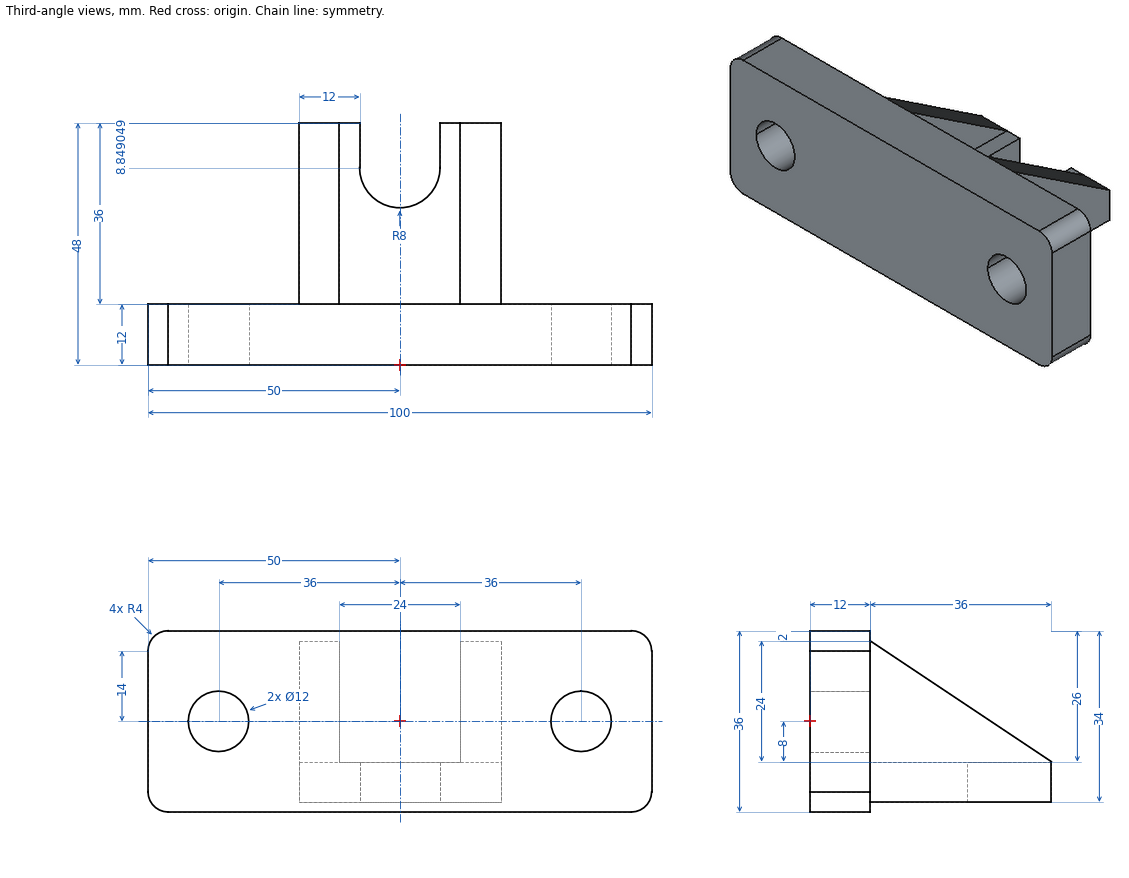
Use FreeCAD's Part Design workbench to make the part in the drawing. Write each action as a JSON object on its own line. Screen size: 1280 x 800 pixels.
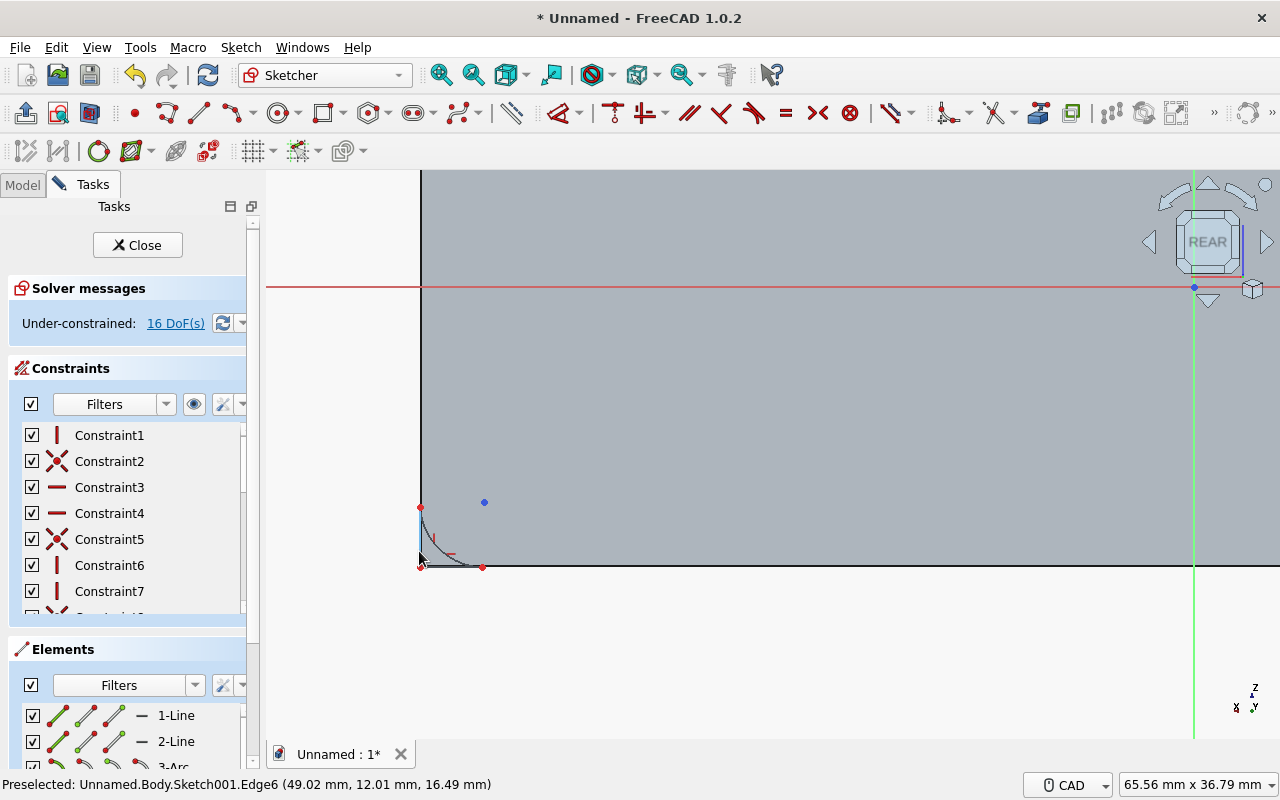
{"action": "left_click", "coordinate": [420, 550]}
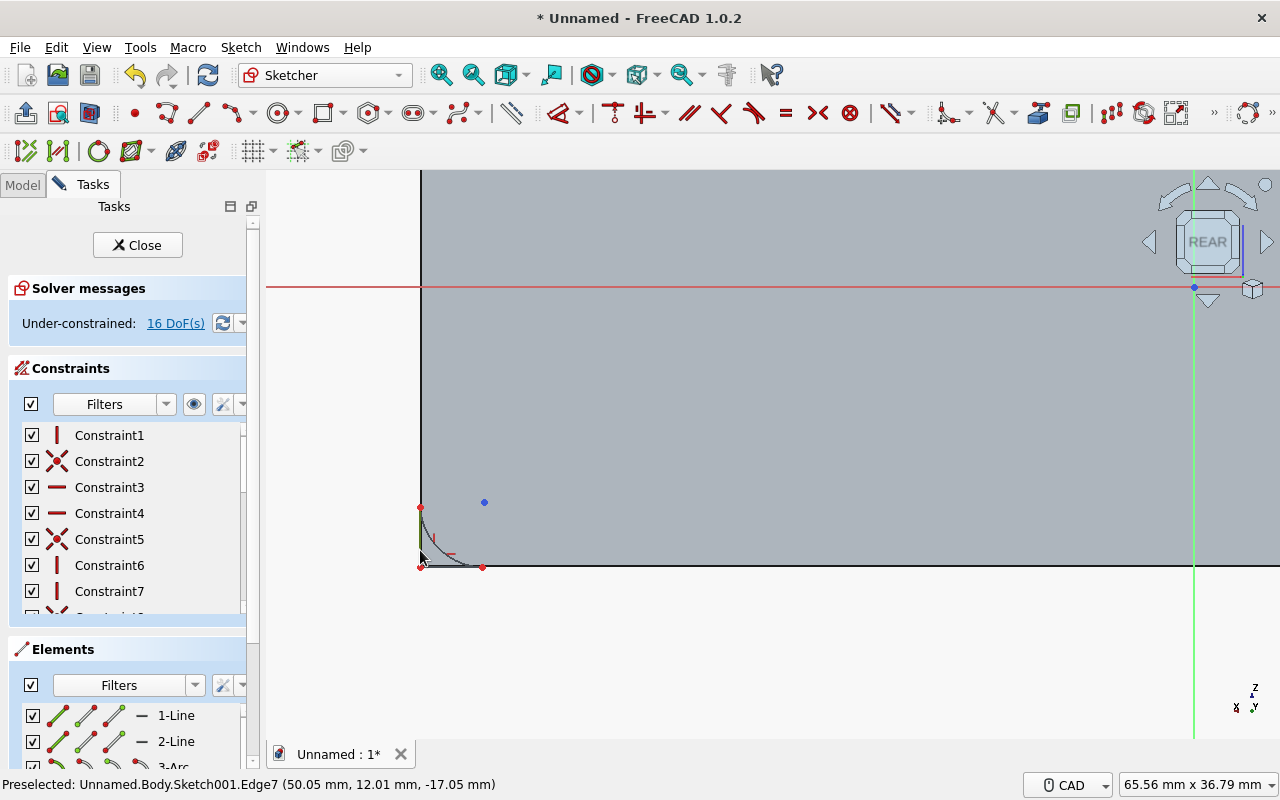
{"action": "left_click", "coordinate": [440, 549]}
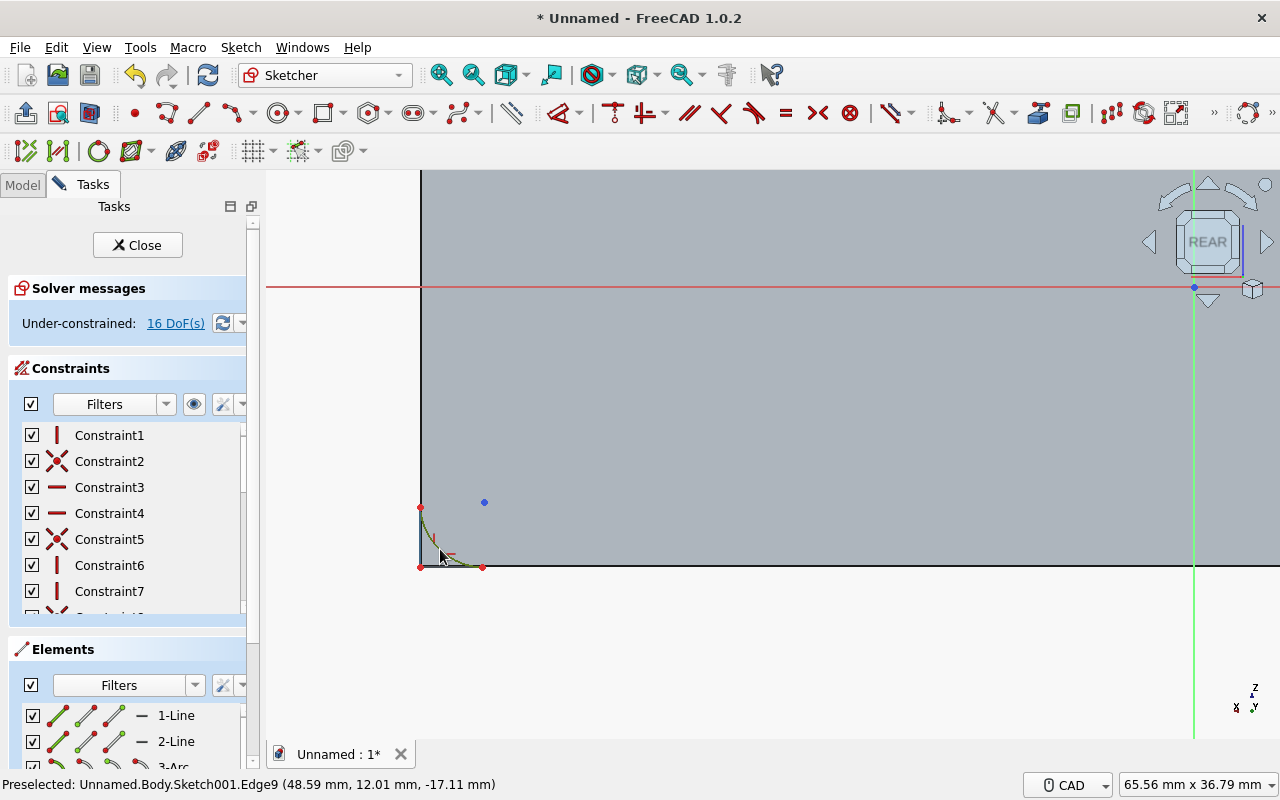
{"action": "left_click", "coordinate": [754, 114]}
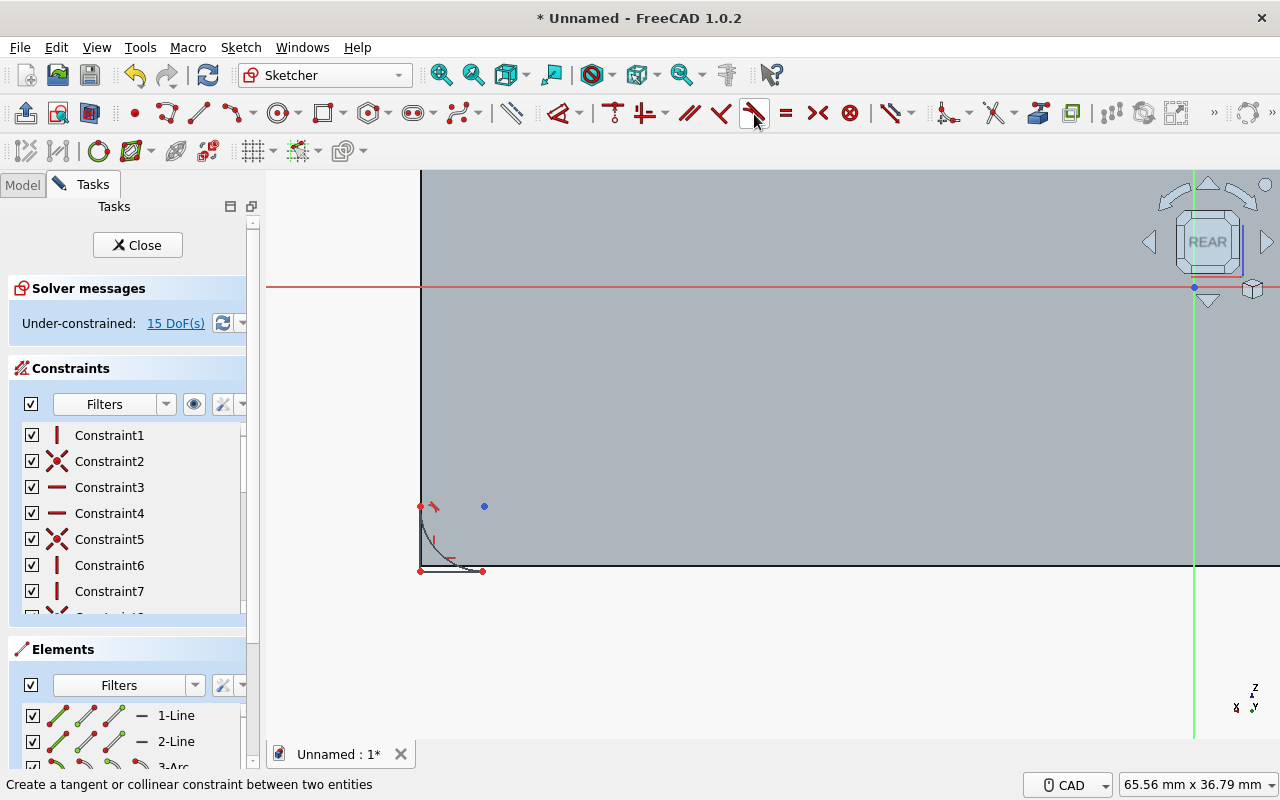
{"action": "left_click", "coordinate": [439, 572]}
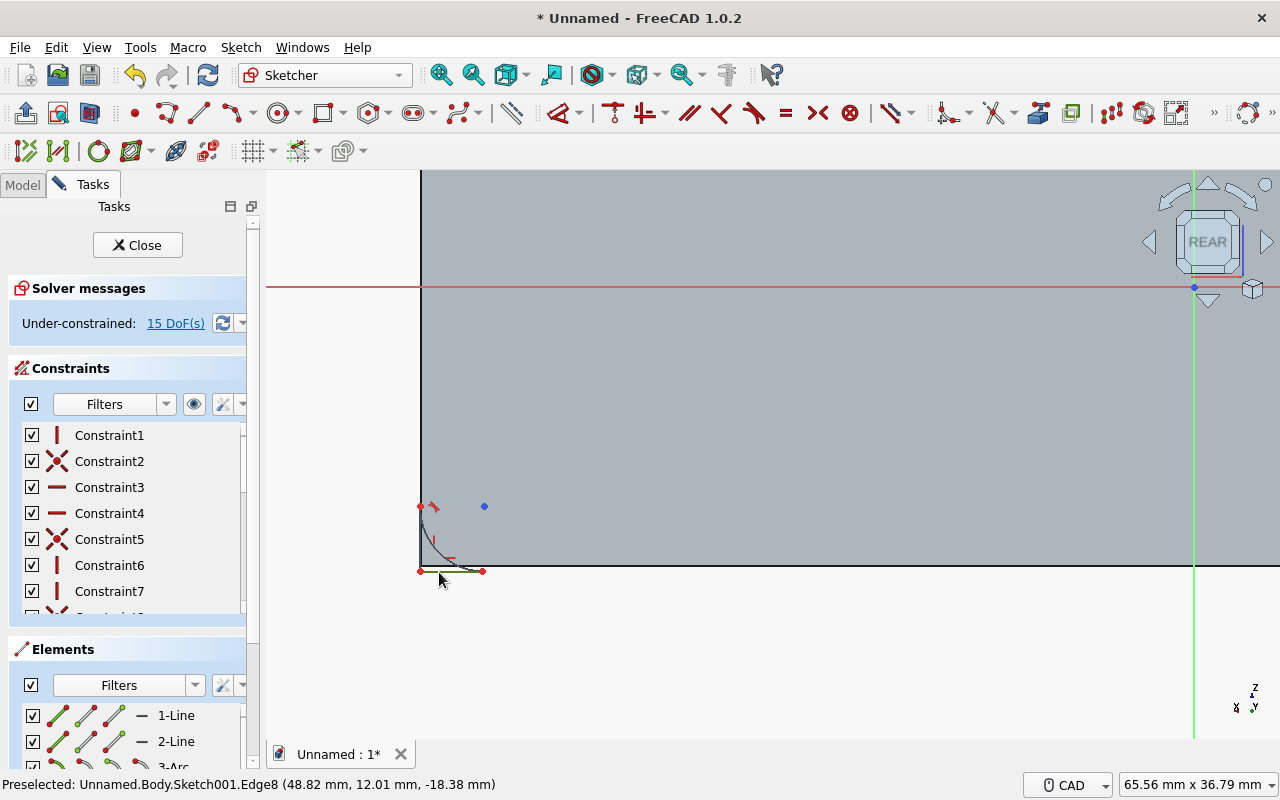
{"action": "left_click", "coordinate": [438, 552]}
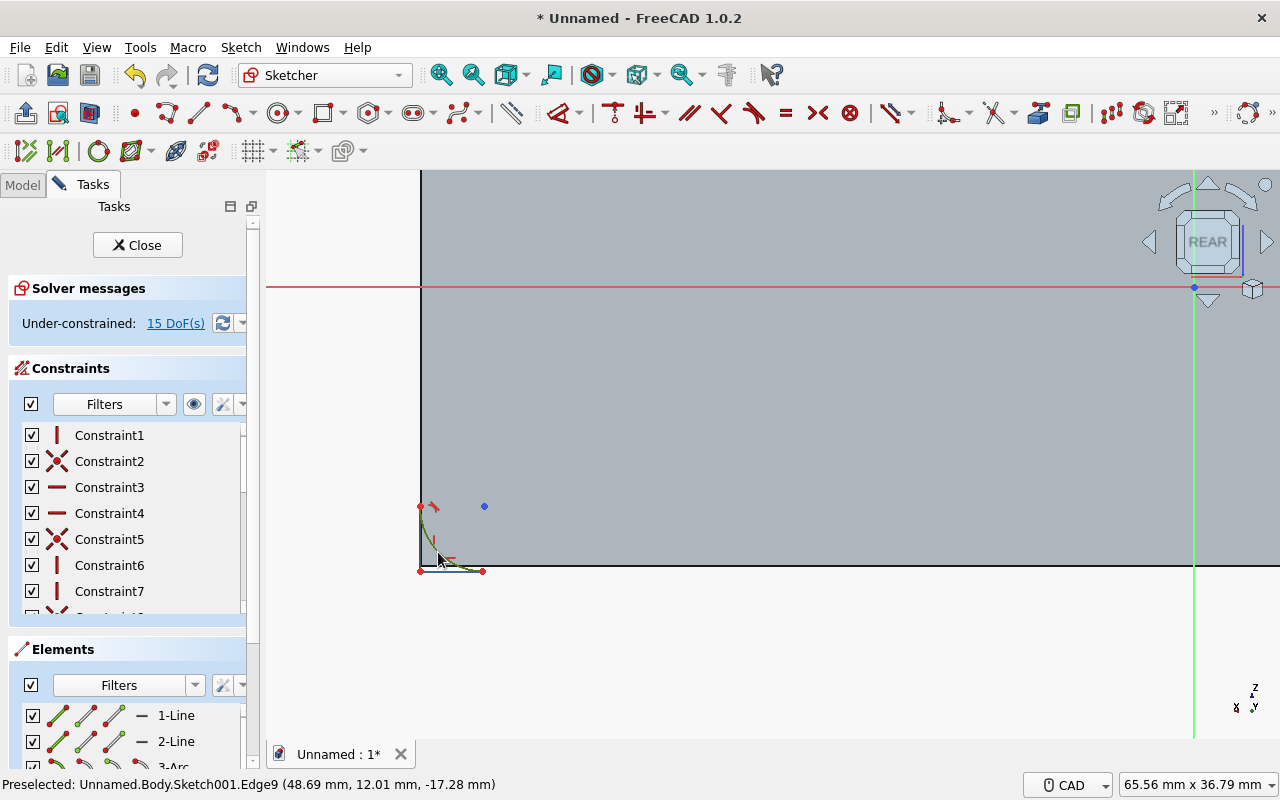
{"action": "left_click", "coordinate": [754, 114]}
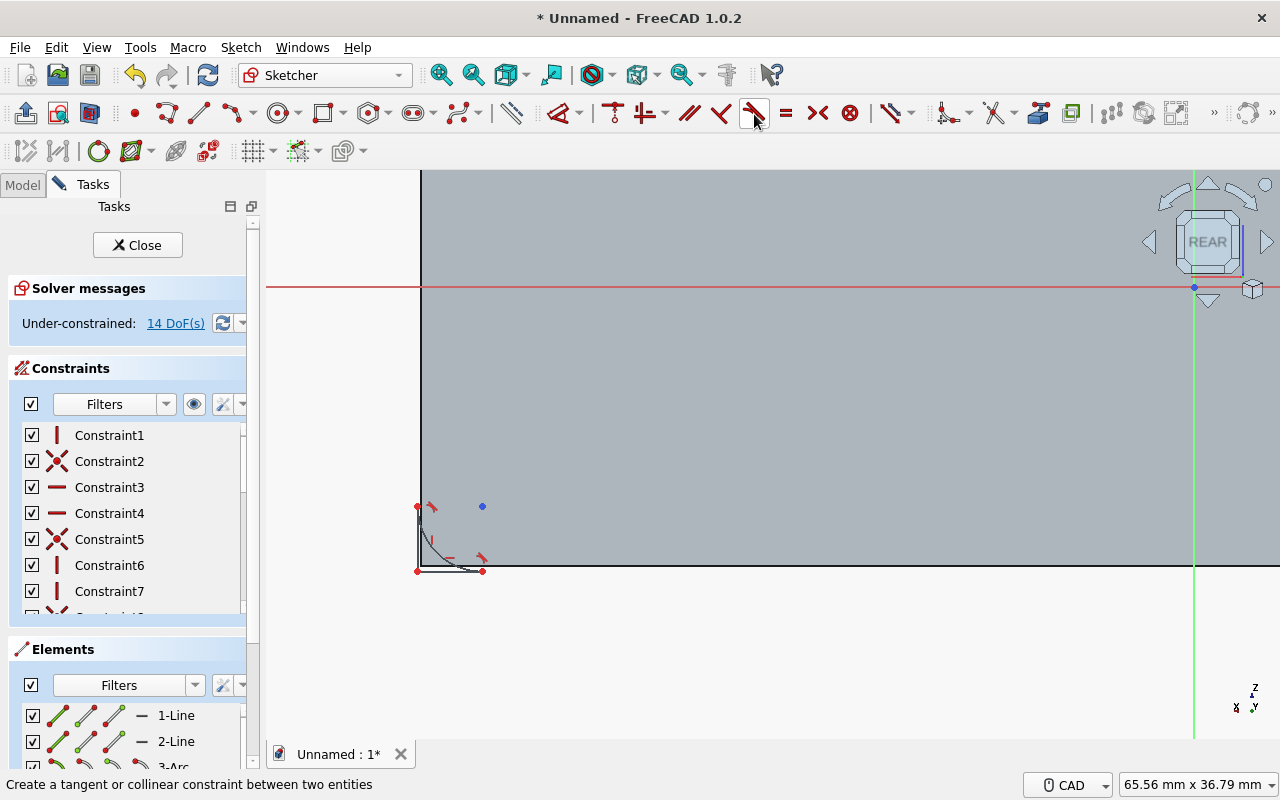
{"action": "scroll", "coordinate": [420, 552], "scroll_direction": "down", "scroll_amount": 5}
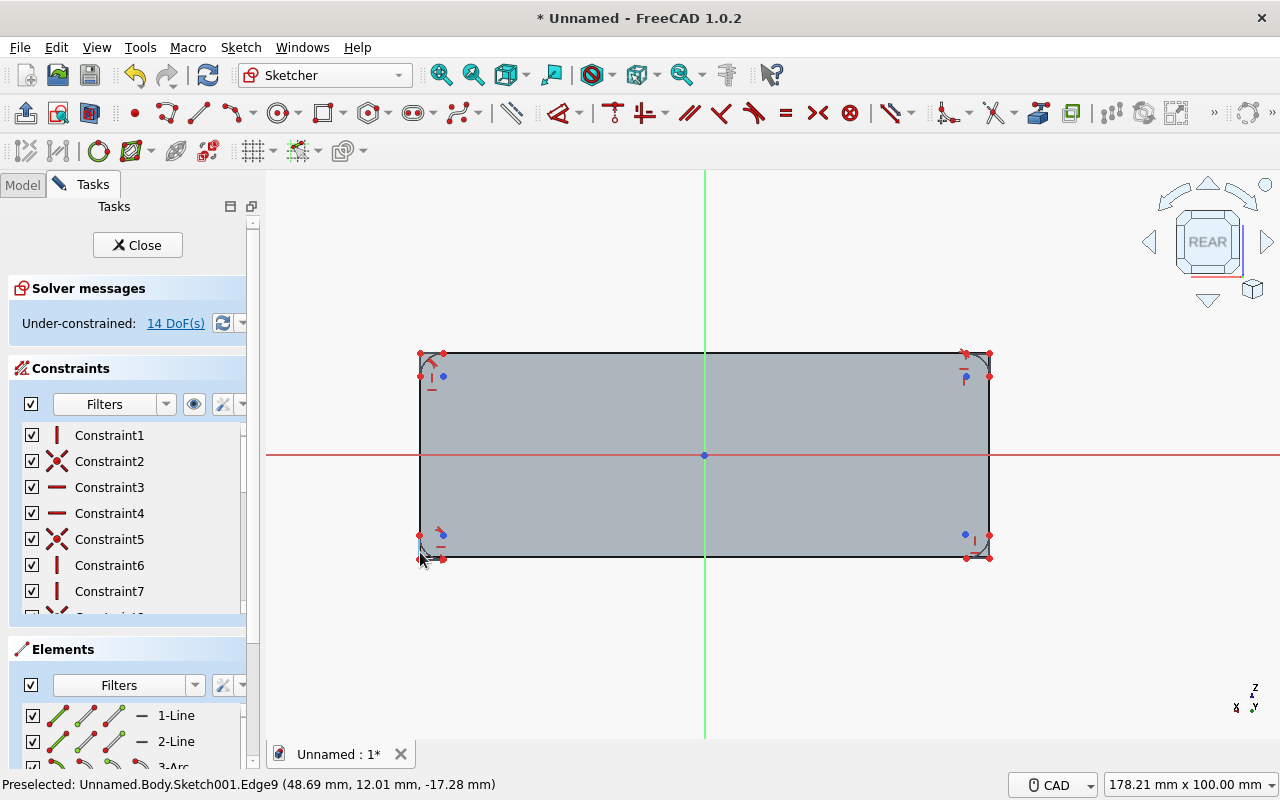
{"action": "scroll", "coordinate": [983, 558], "scroll_direction": "up", "scroll_amount": 5}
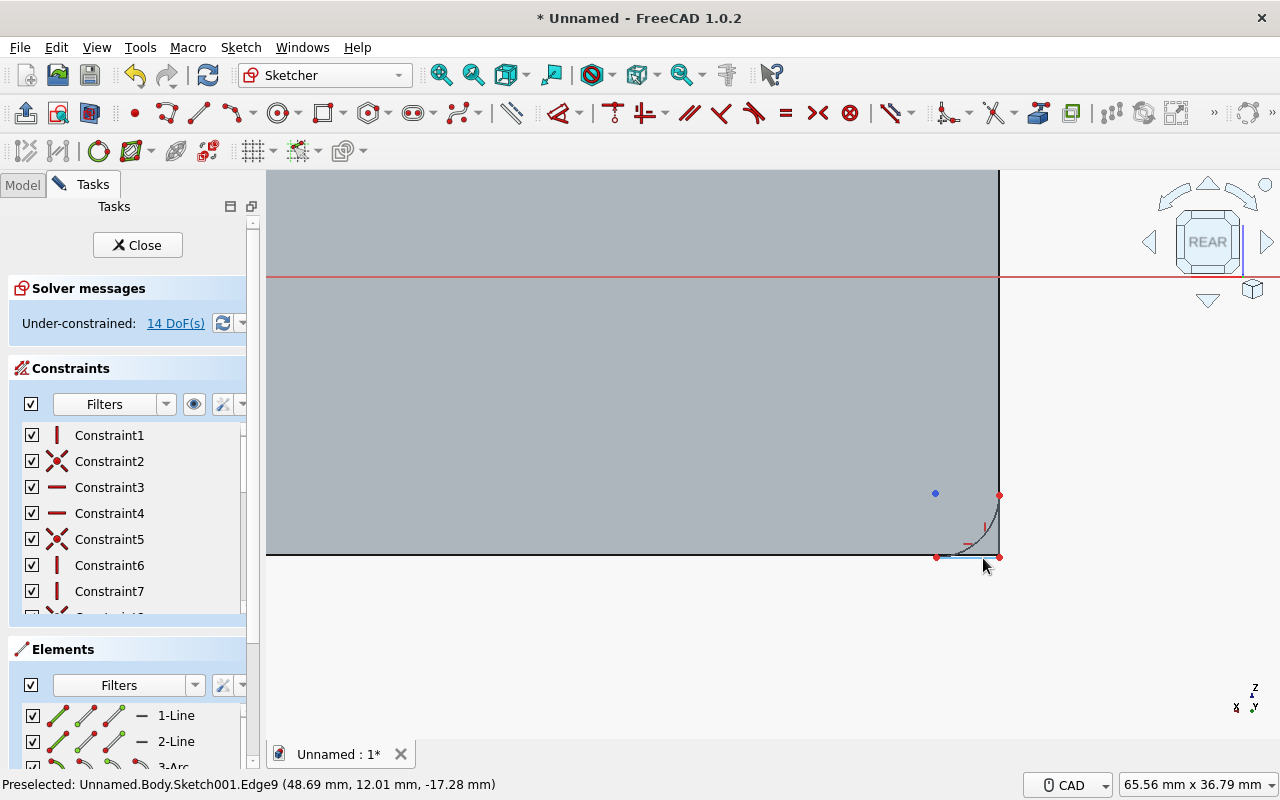
{"action": "left_click", "coordinate": [981, 558]}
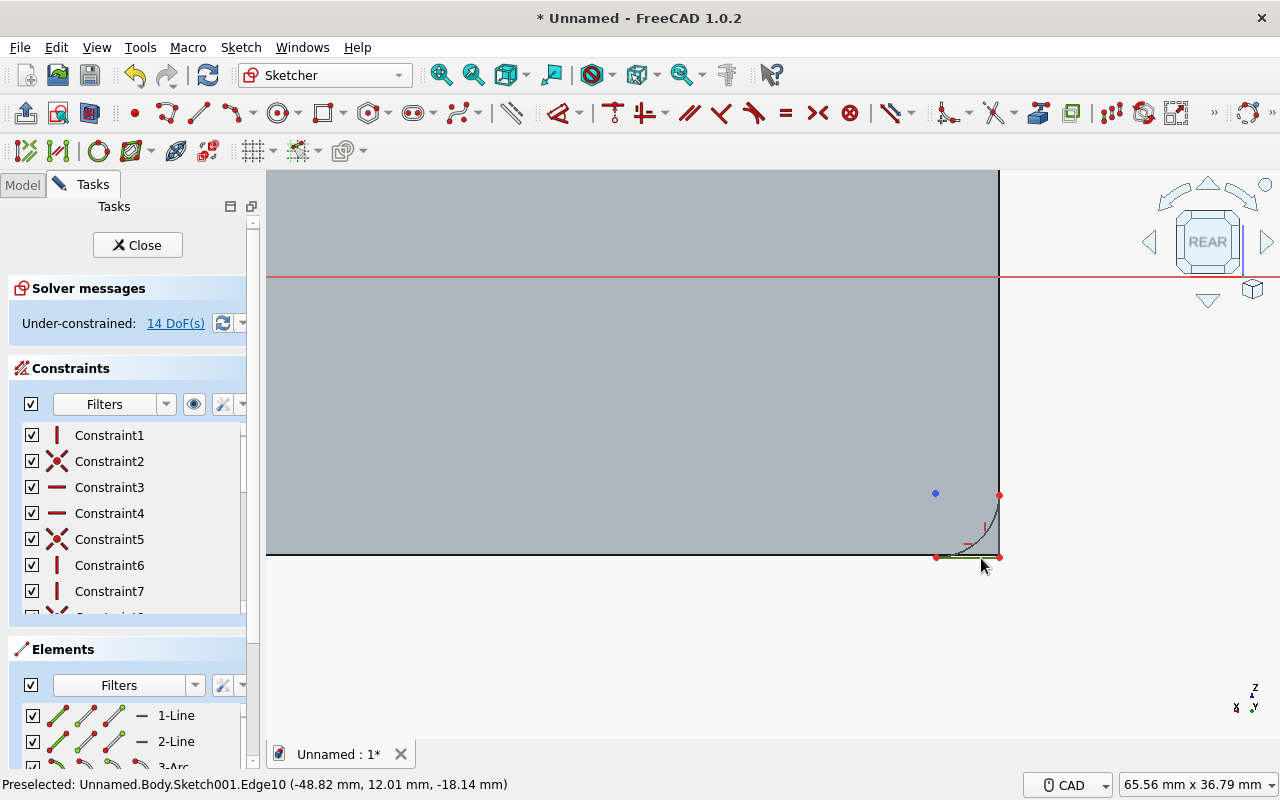
{"action": "left_click", "coordinate": [981, 539]}